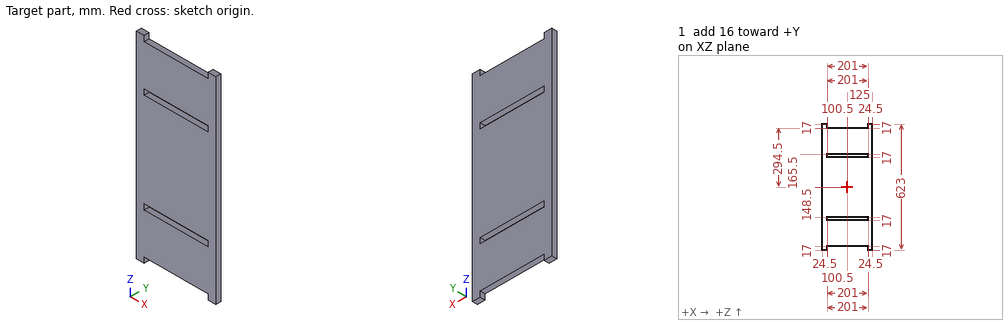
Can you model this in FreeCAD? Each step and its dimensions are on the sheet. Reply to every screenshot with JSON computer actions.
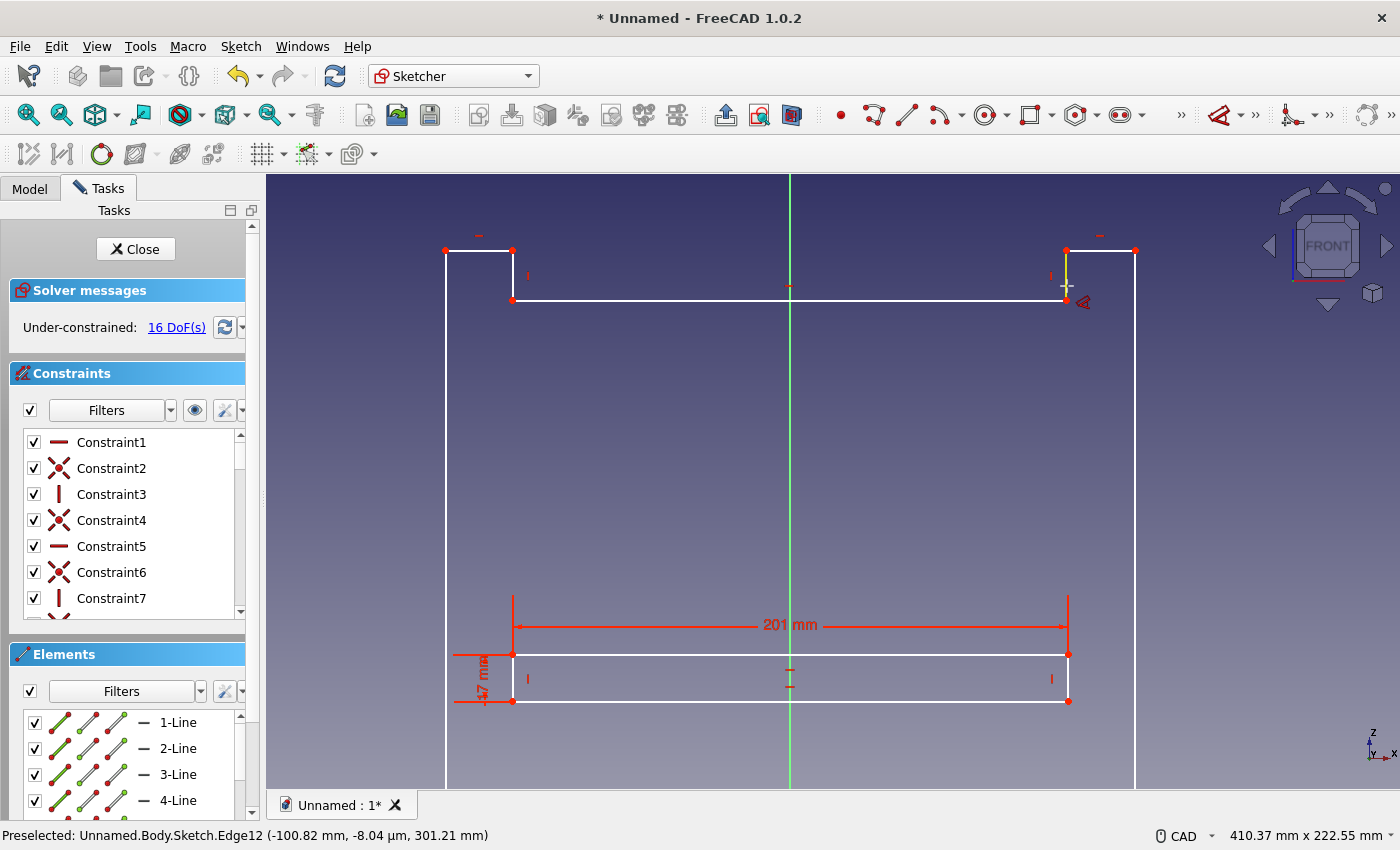
{"action": "left_click", "coordinate": [1066, 286]}
{"action": "left_click", "coordinate": [1100, 276]}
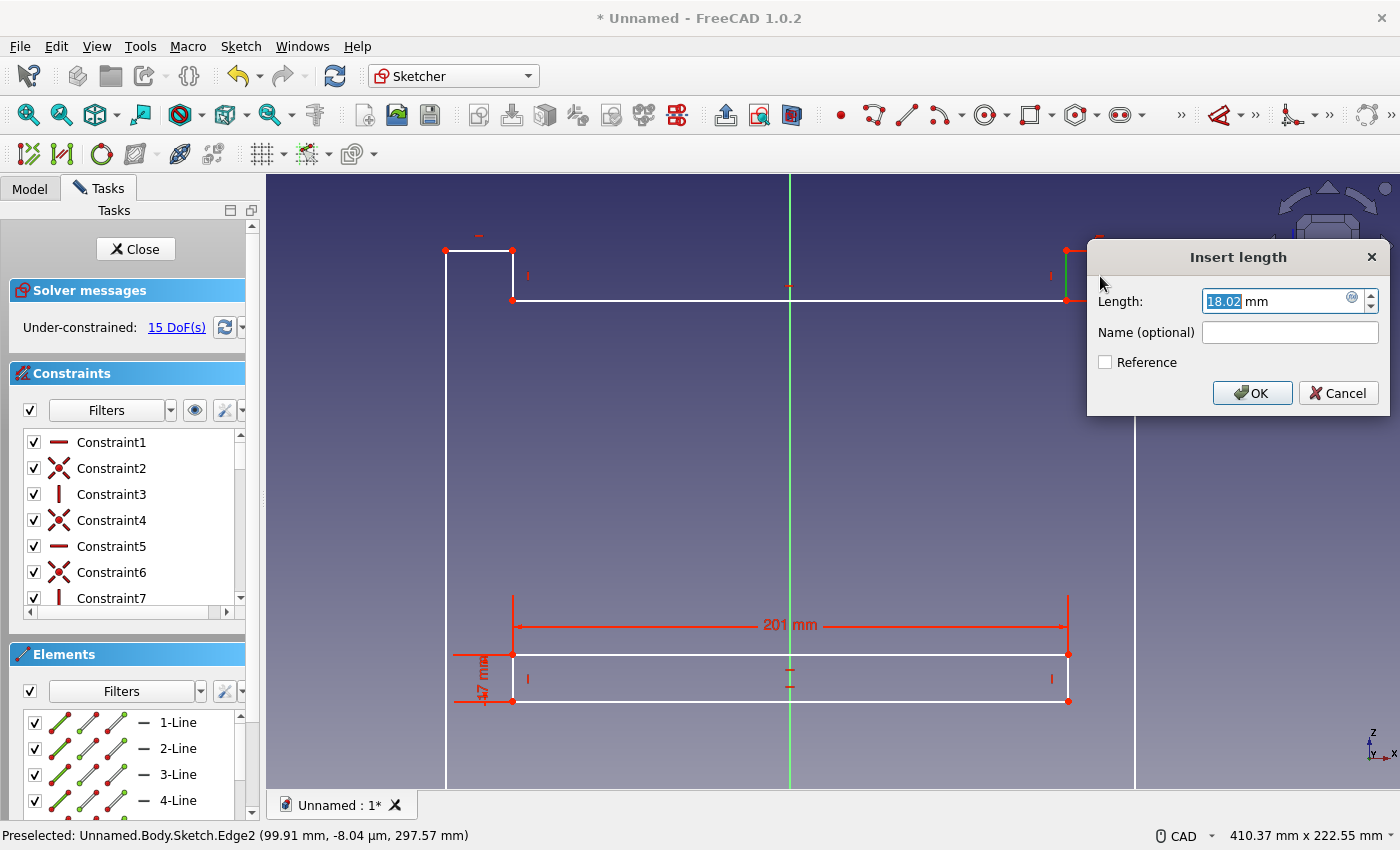
{"action": "type", "text": "17"}
{"action": "key", "text": "Return"}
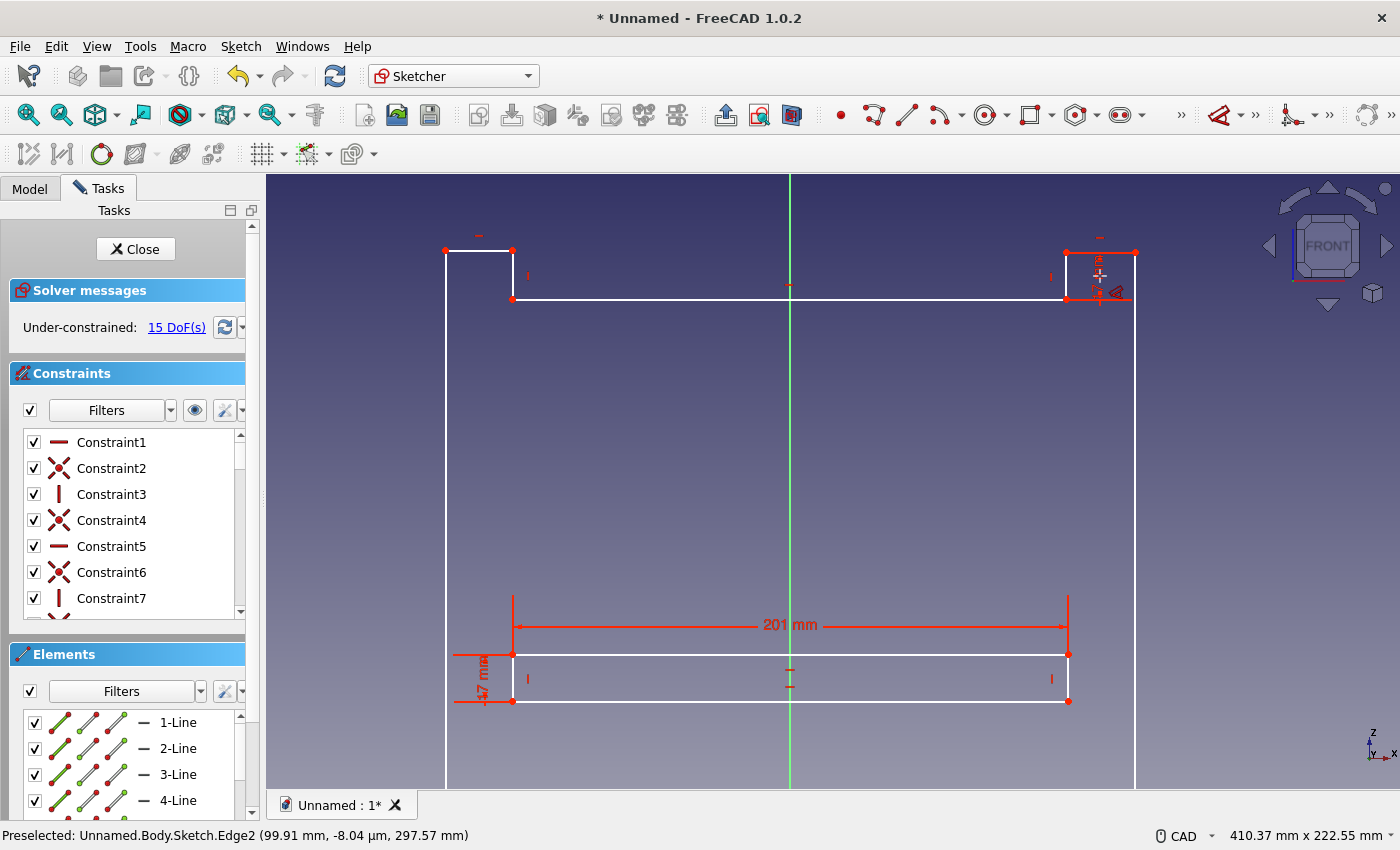
{"action": "scroll", "coordinate": [756, 276], "scroll_direction": "down", "scroll_amount": 7}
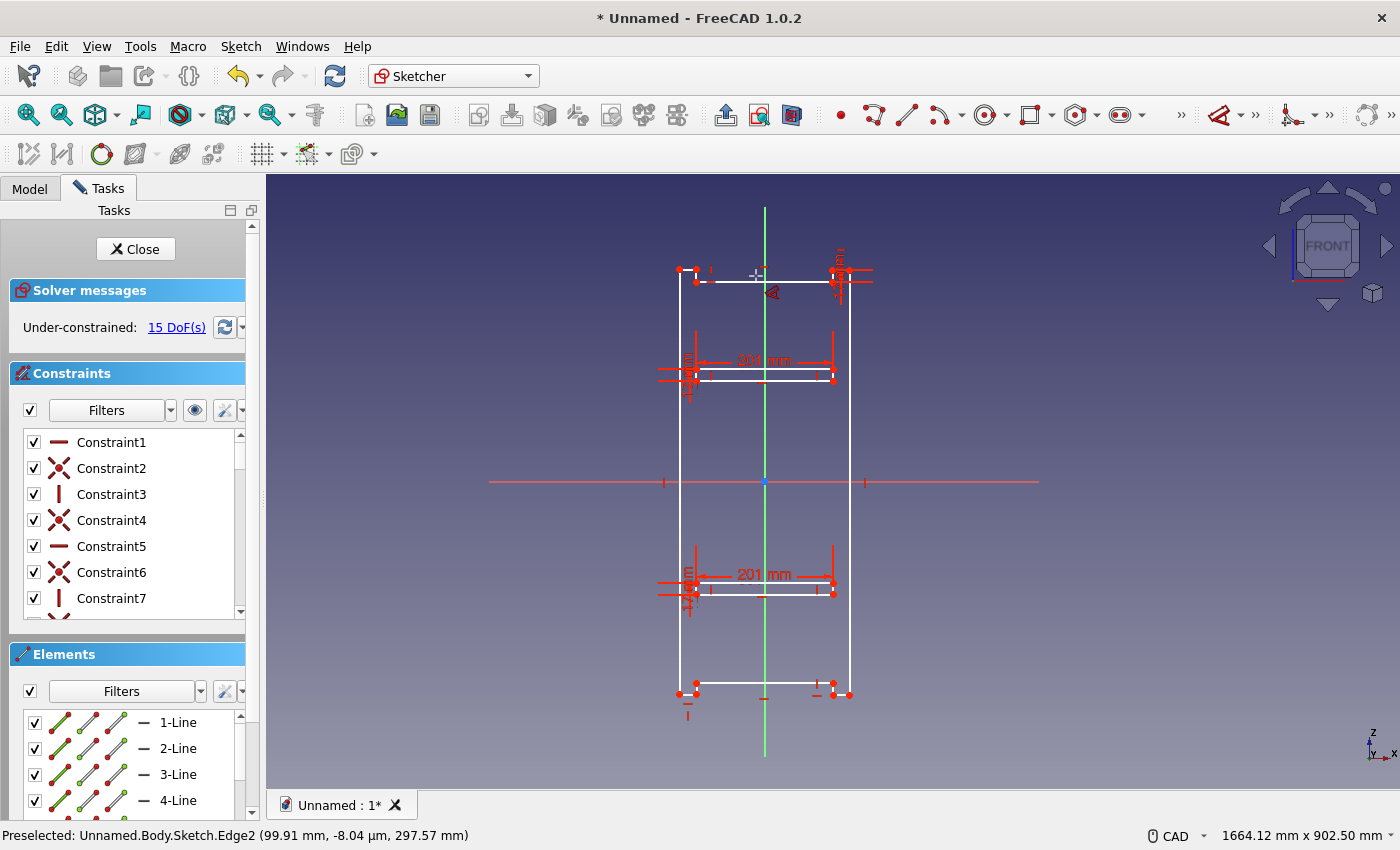
{"action": "scroll", "coordinate": [833, 692], "scroll_direction": "up", "scroll_amount": 7}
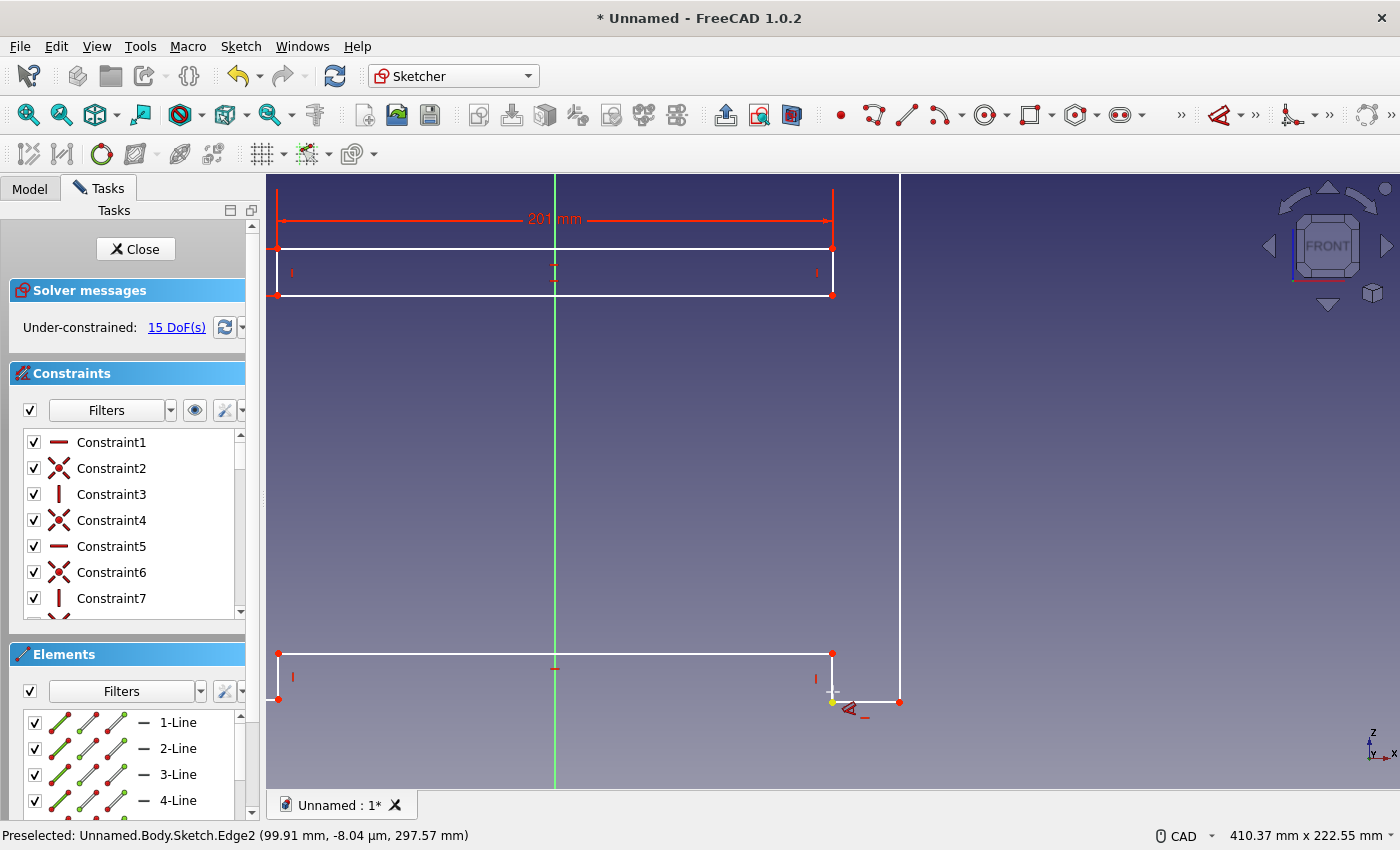
{"action": "left_click", "coordinate": [832, 688]}
{"action": "left_click", "coordinate": [866, 678]}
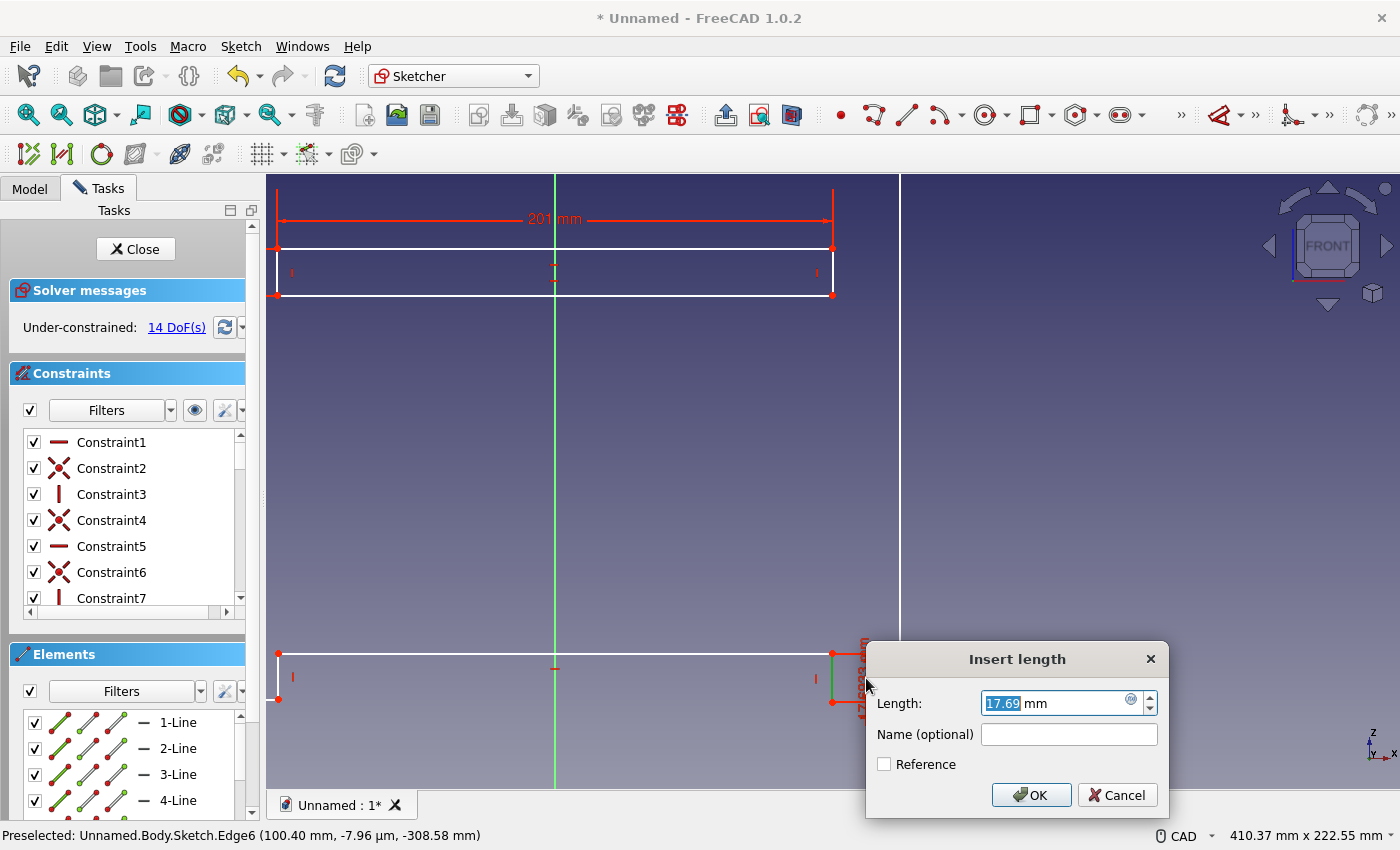
{"action": "type", "text": "17"}
{"action": "key", "text": "Return"}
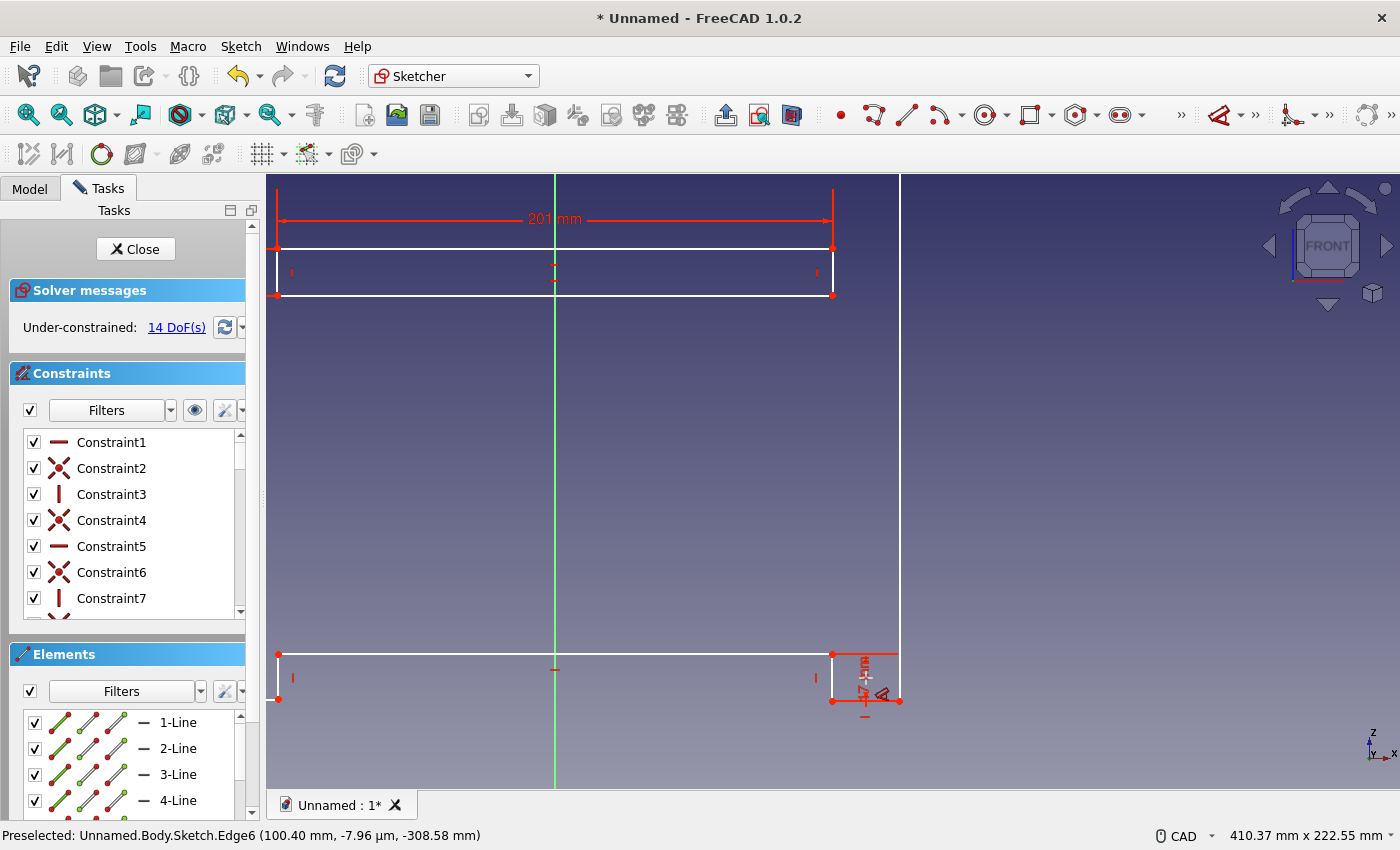
{"action": "scroll", "coordinate": [833, 693], "scroll_direction": "down", "scroll_amount": 7}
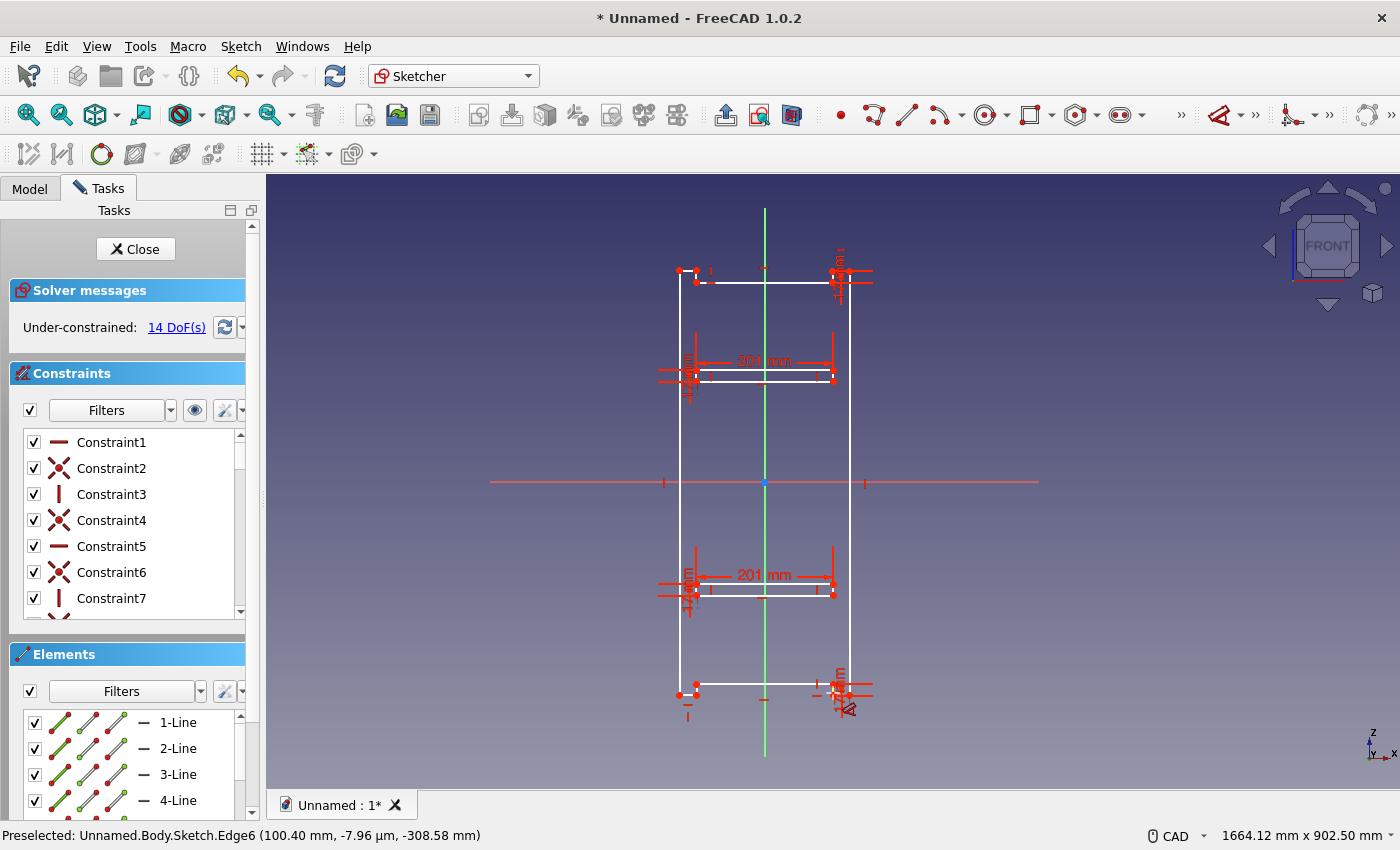
{"action": "scroll", "coordinate": [697, 687], "scroll_direction": "up", "scroll_amount": 8}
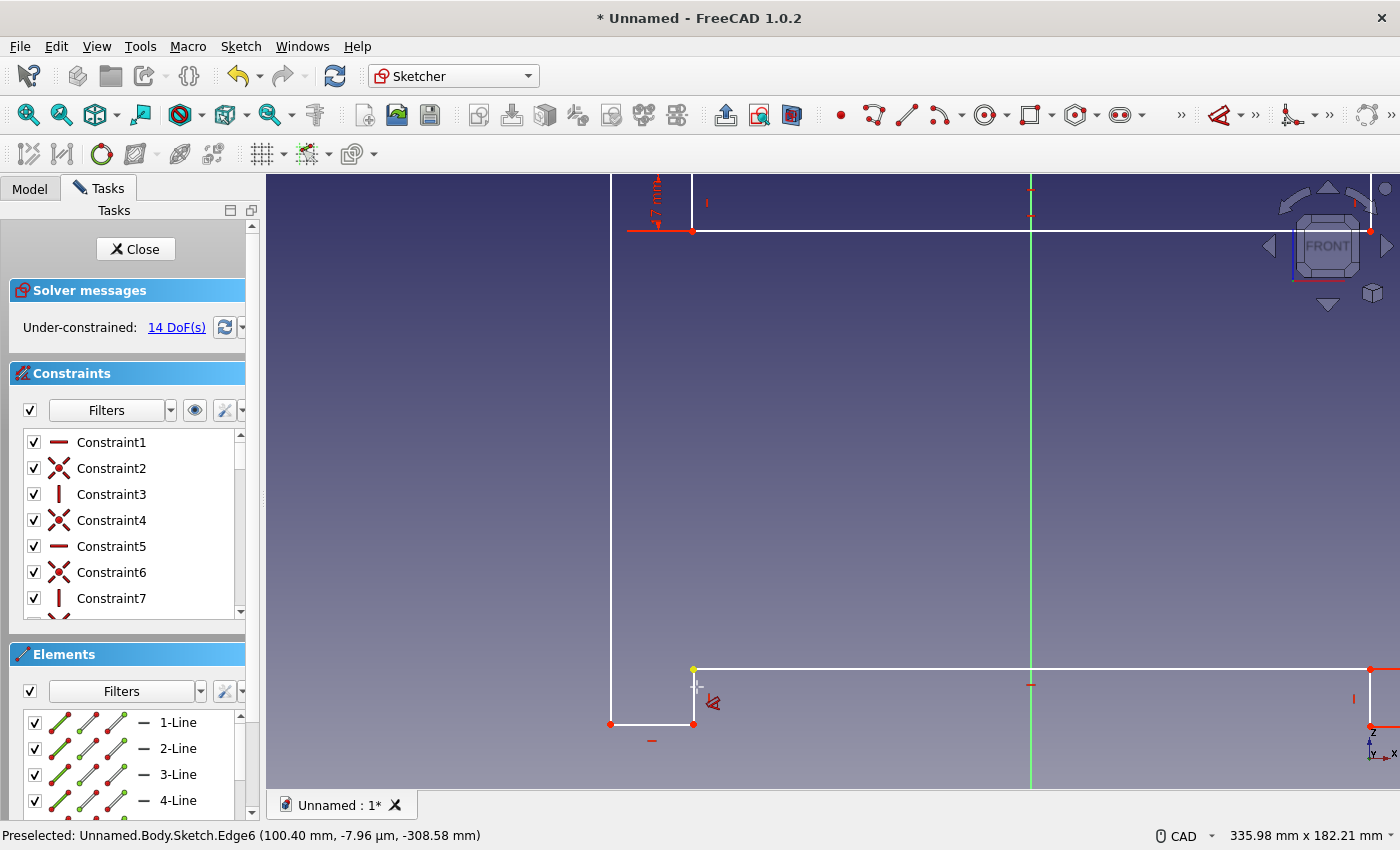
{"action": "left_click", "coordinate": [694, 686]}
{"action": "left_click", "coordinate": [660, 697]}